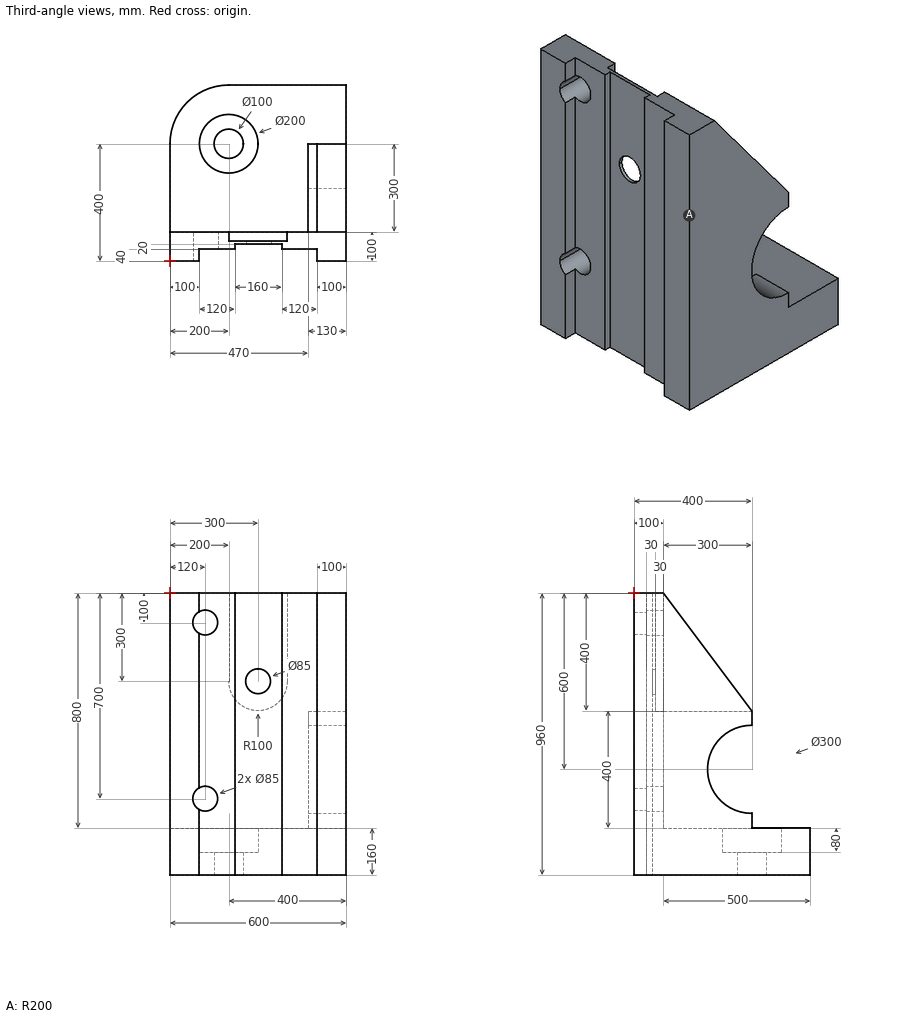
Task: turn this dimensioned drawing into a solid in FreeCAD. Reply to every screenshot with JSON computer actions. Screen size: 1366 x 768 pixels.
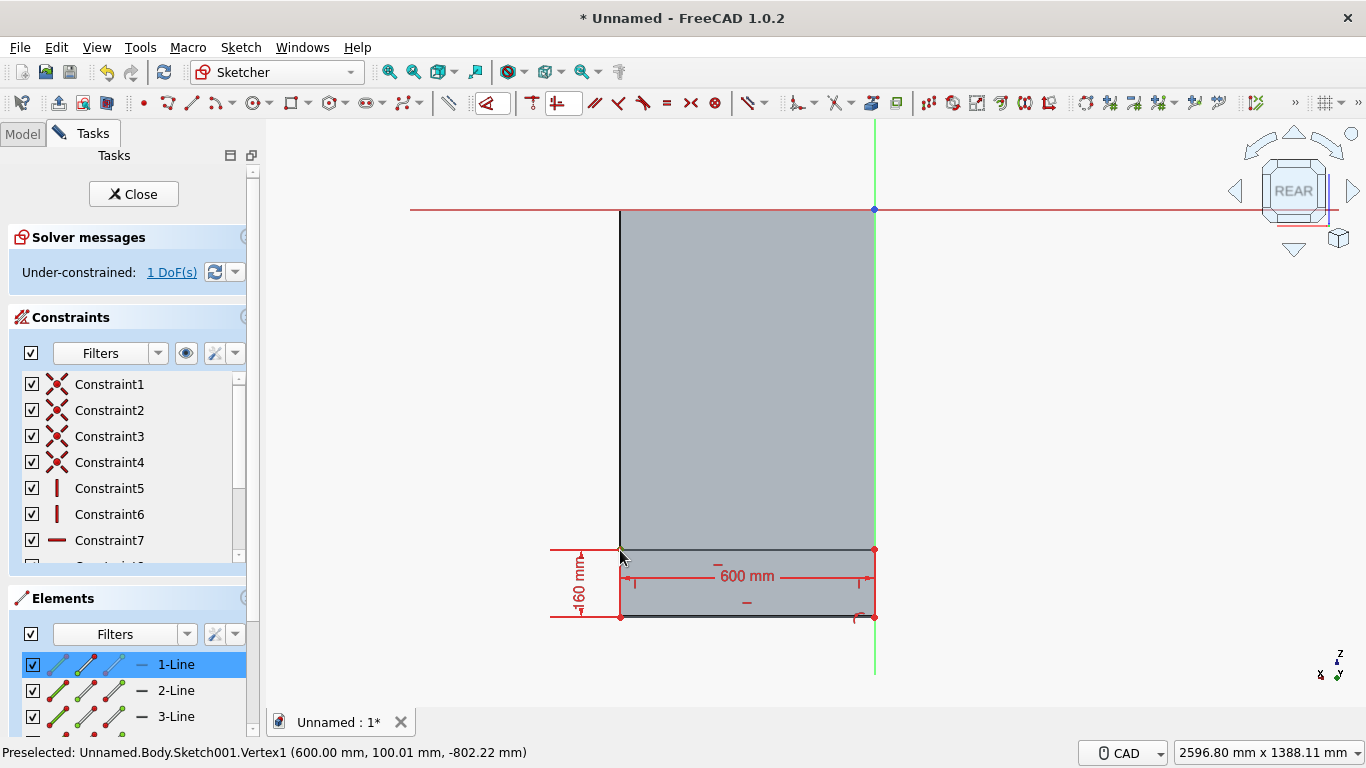
{"action": "key", "text": "i"}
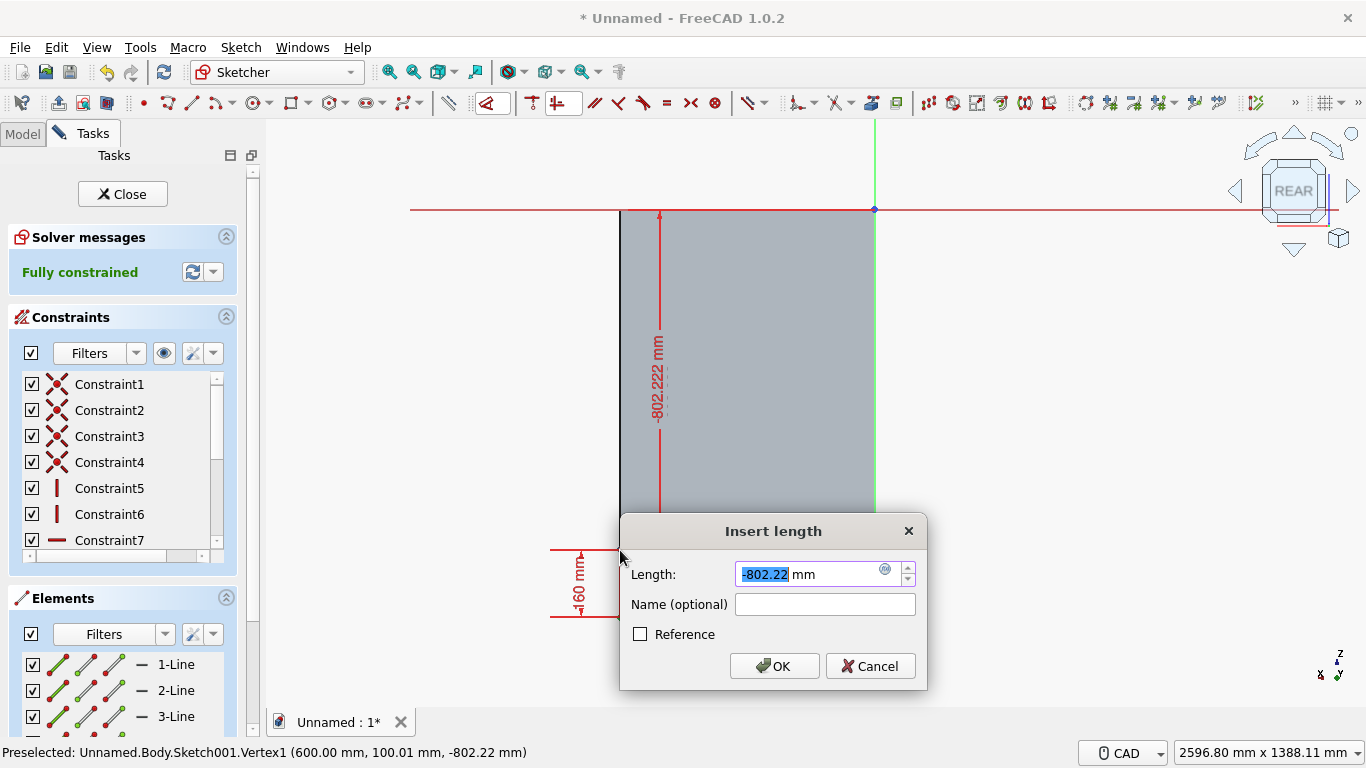
{"action": "type", "text": "-800"}
{"action": "key", "text": "Return"}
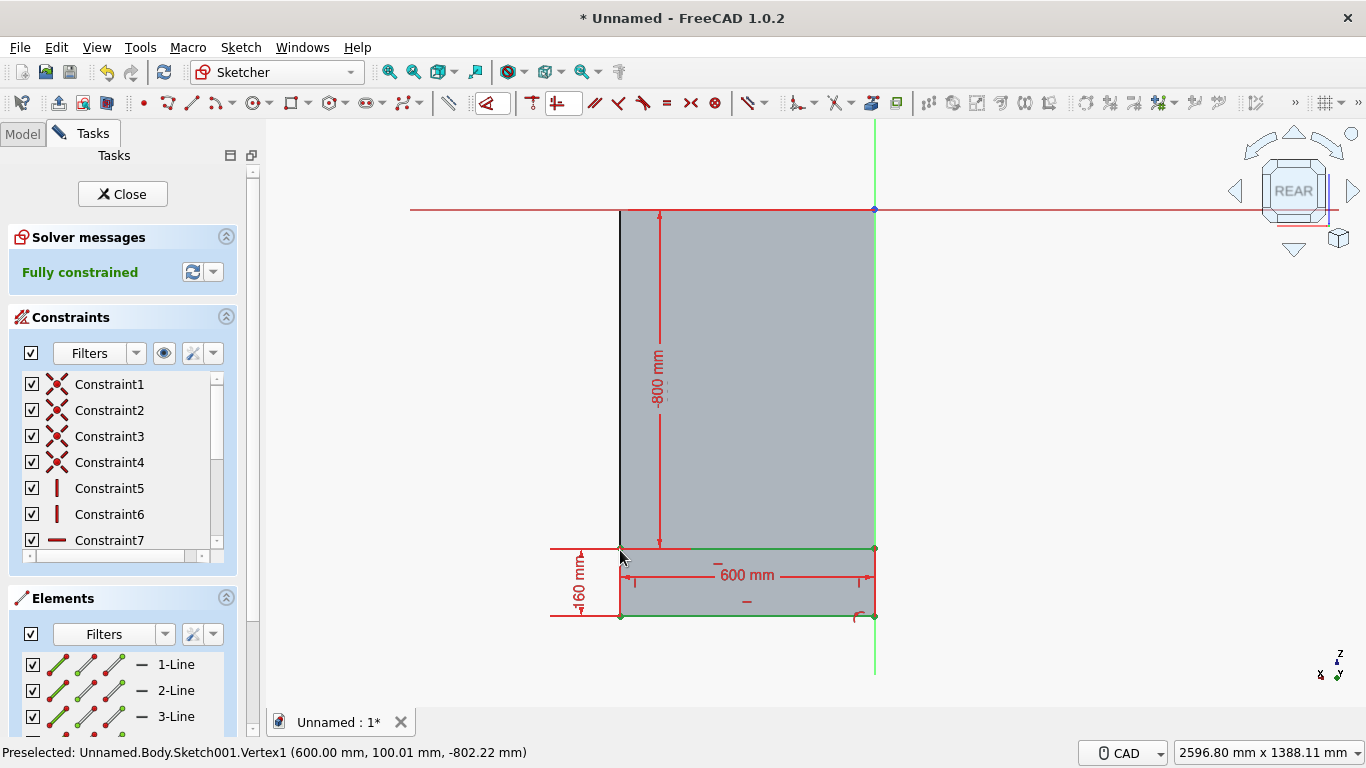
{"action": "left_click", "coordinate": [123, 194]}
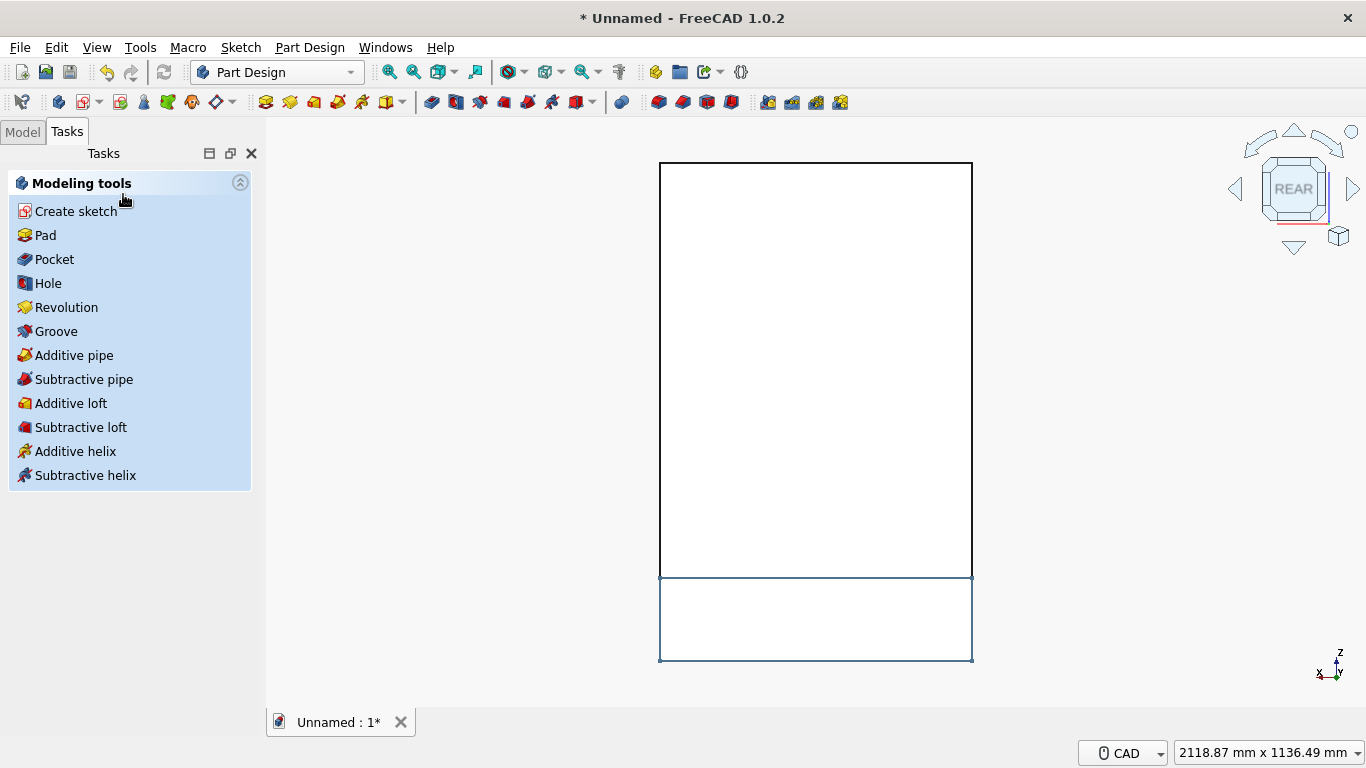
{"action": "left_click", "coordinate": [266, 102]}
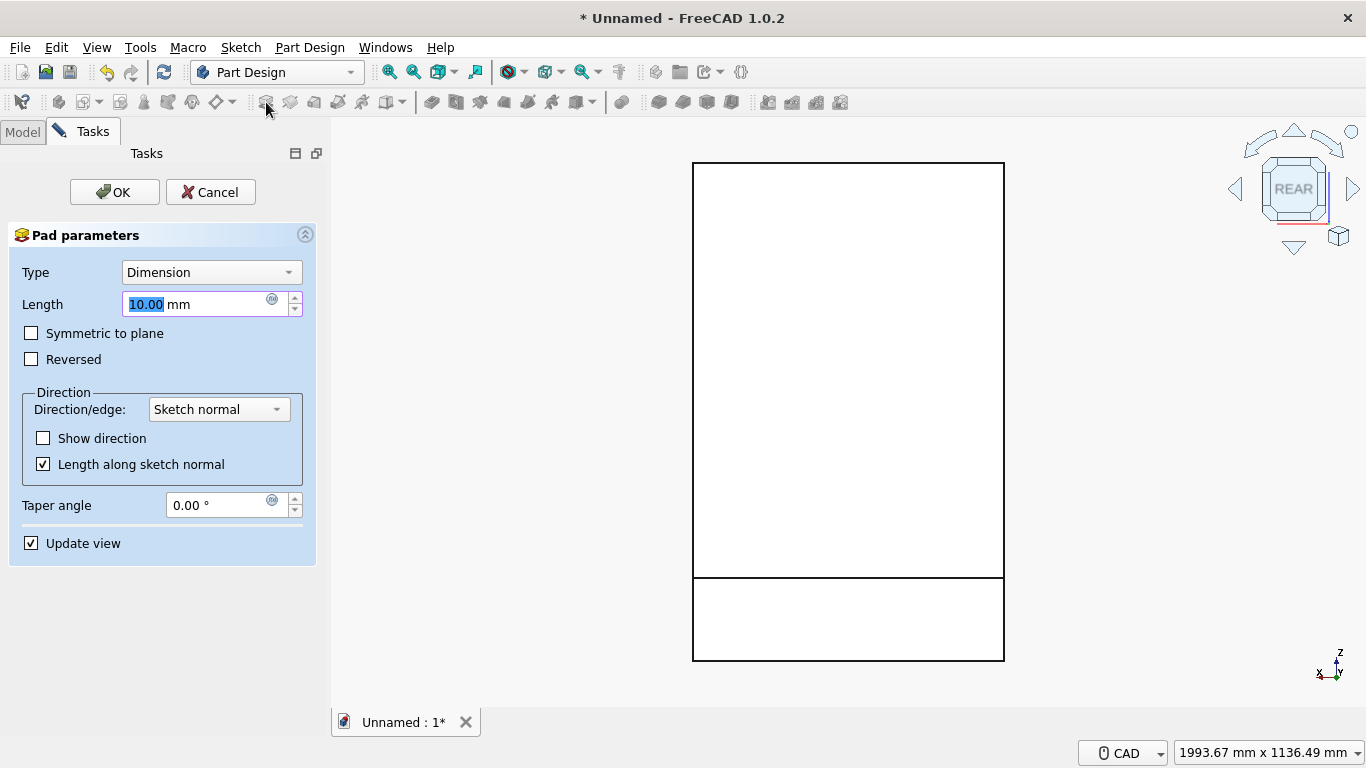
{"action": "type", "text": "500"}
{"action": "key", "text": "Tab"}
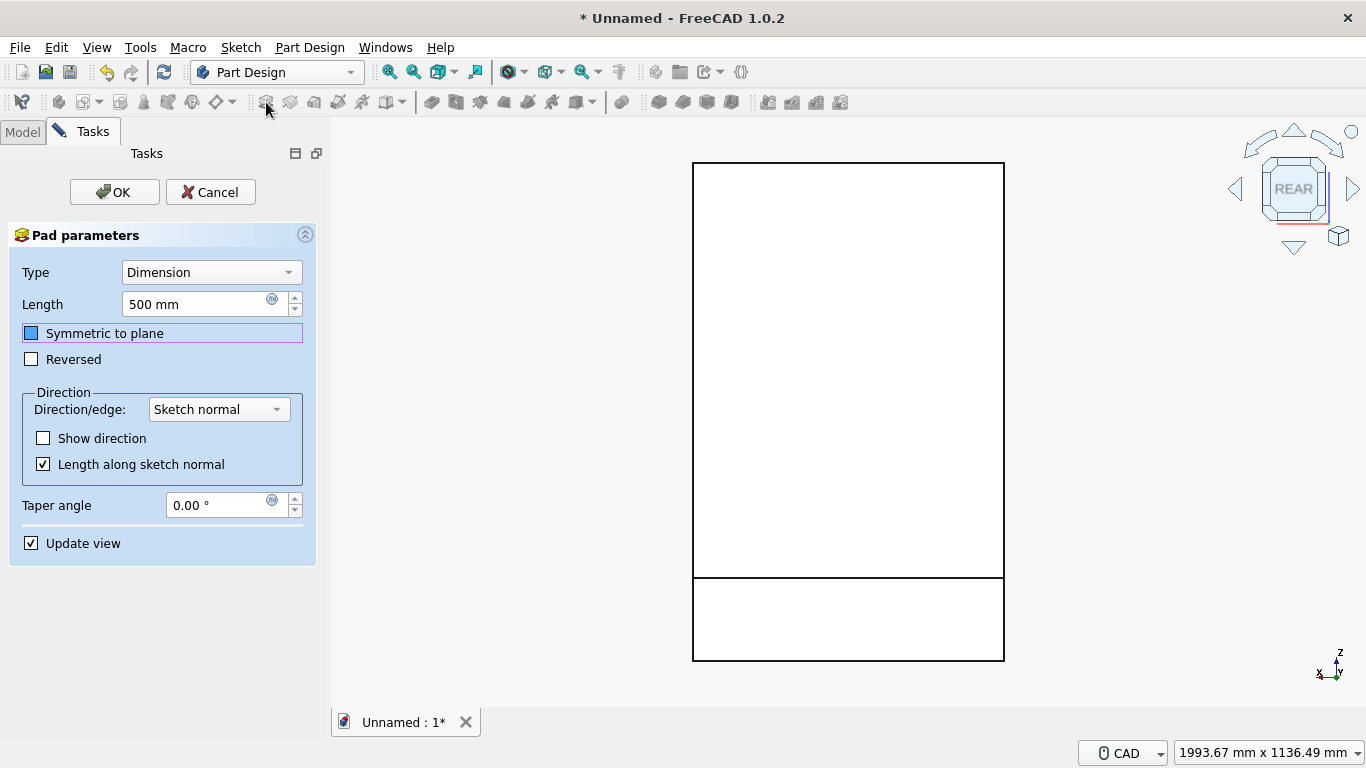
{"action": "left_click", "coordinate": [115, 192]}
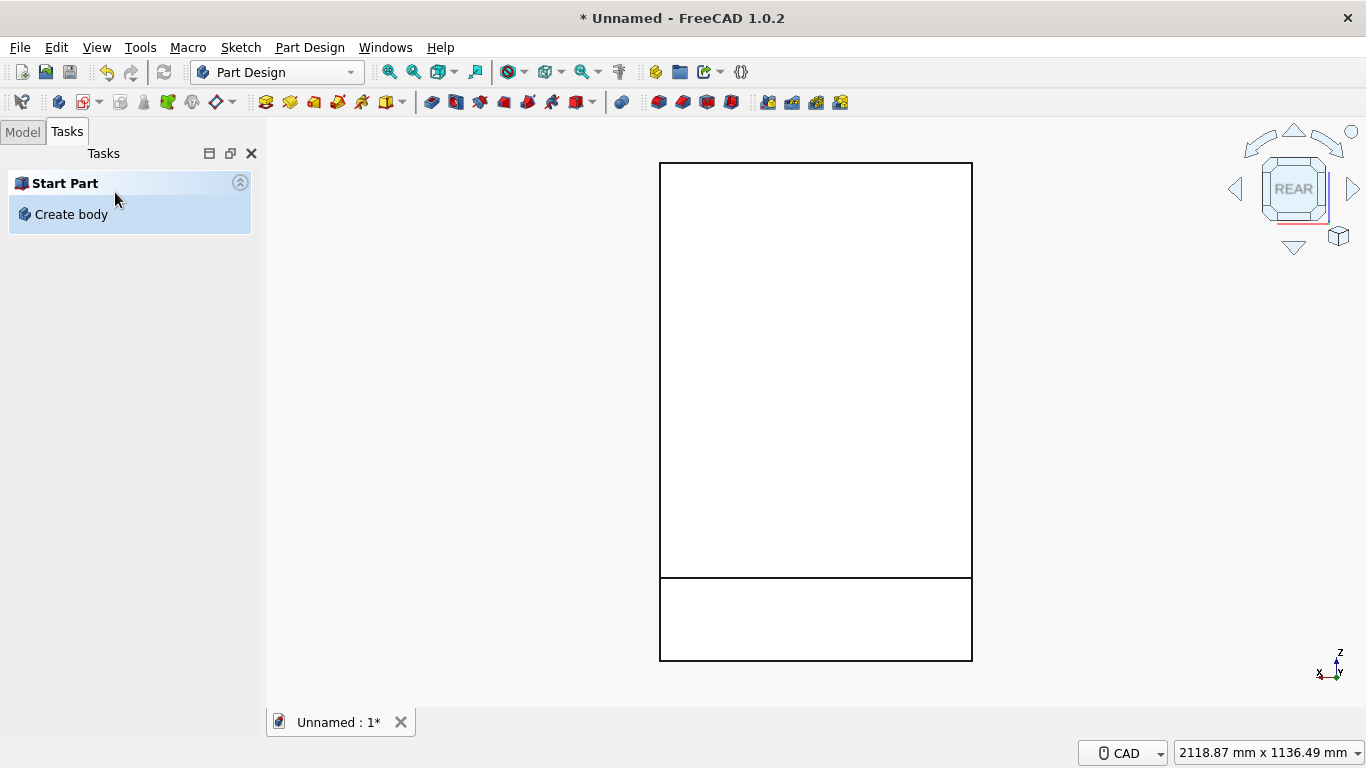
{"action": "left_click", "coordinate": [972, 619]}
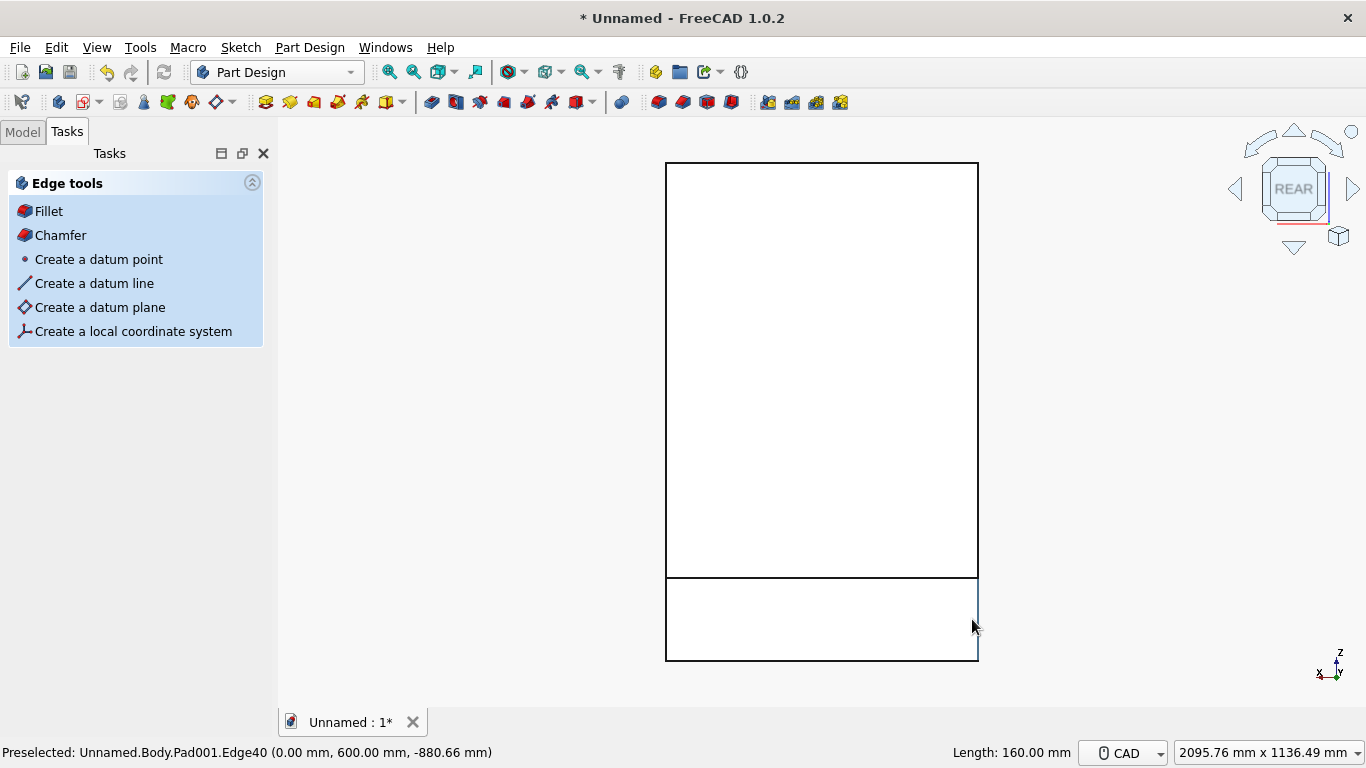
{"action": "left_click", "coordinate": [660, 102]}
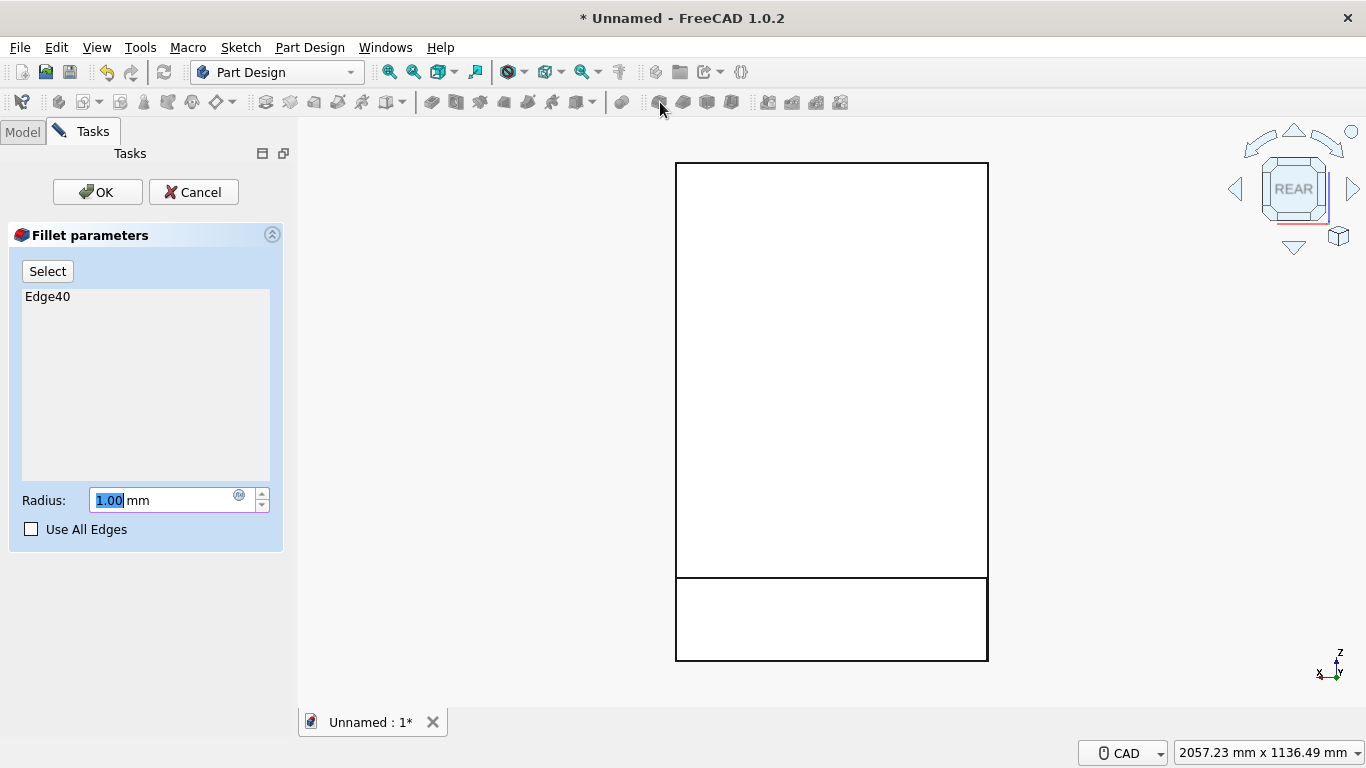
{"action": "type", "text": "200"}
{"action": "key", "text": "Tab"}